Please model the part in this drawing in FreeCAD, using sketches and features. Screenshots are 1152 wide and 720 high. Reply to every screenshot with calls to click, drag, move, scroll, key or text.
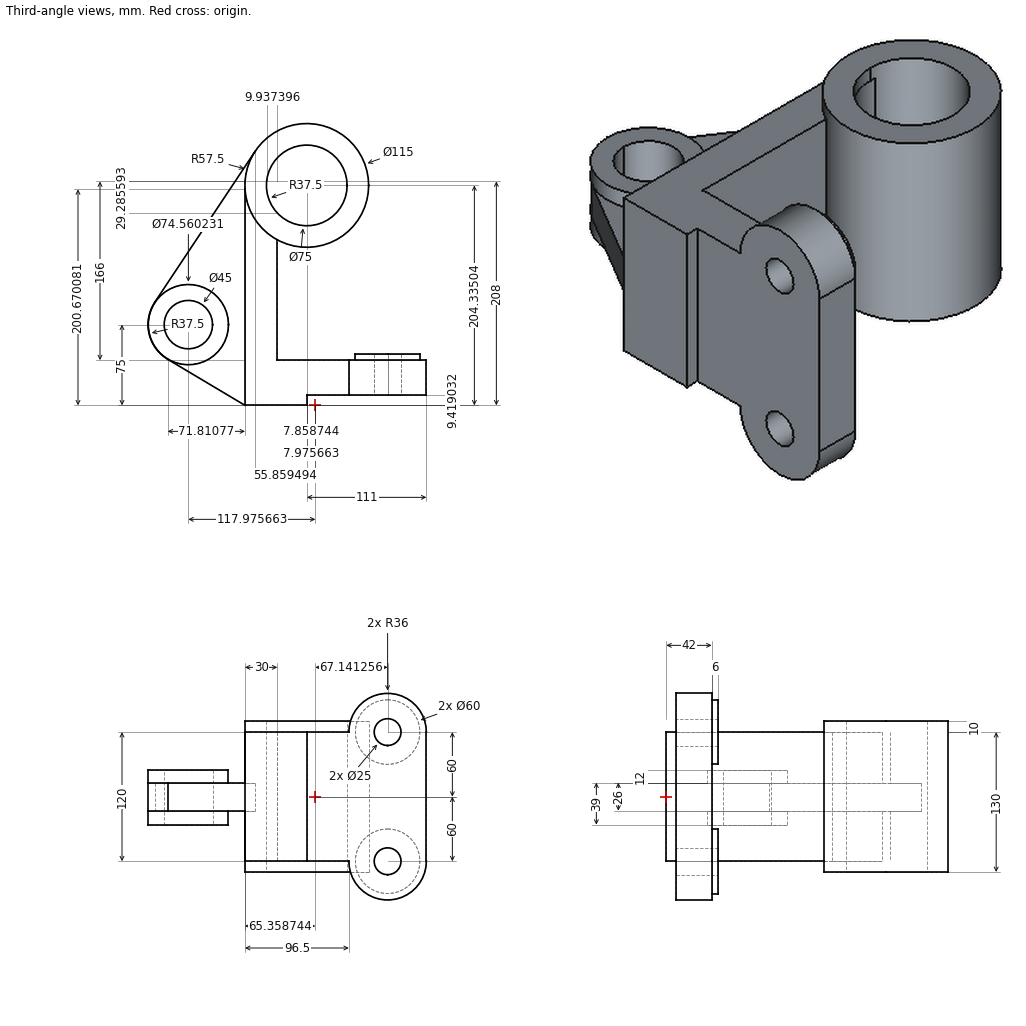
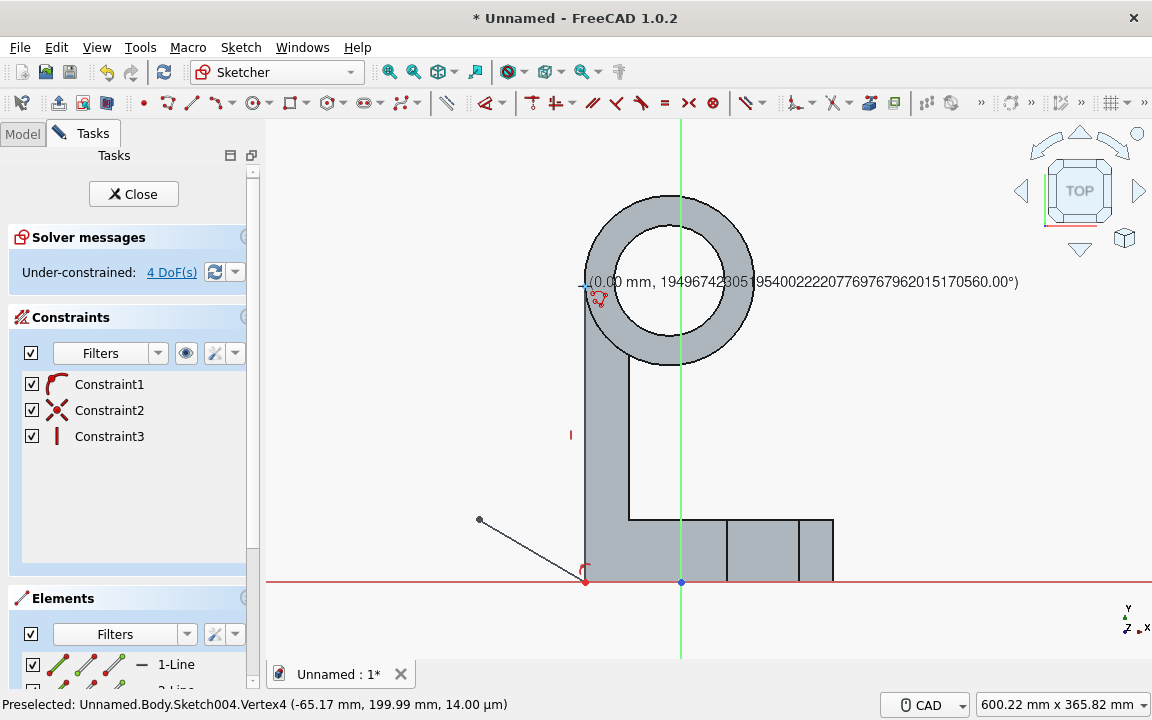
click(192, 104)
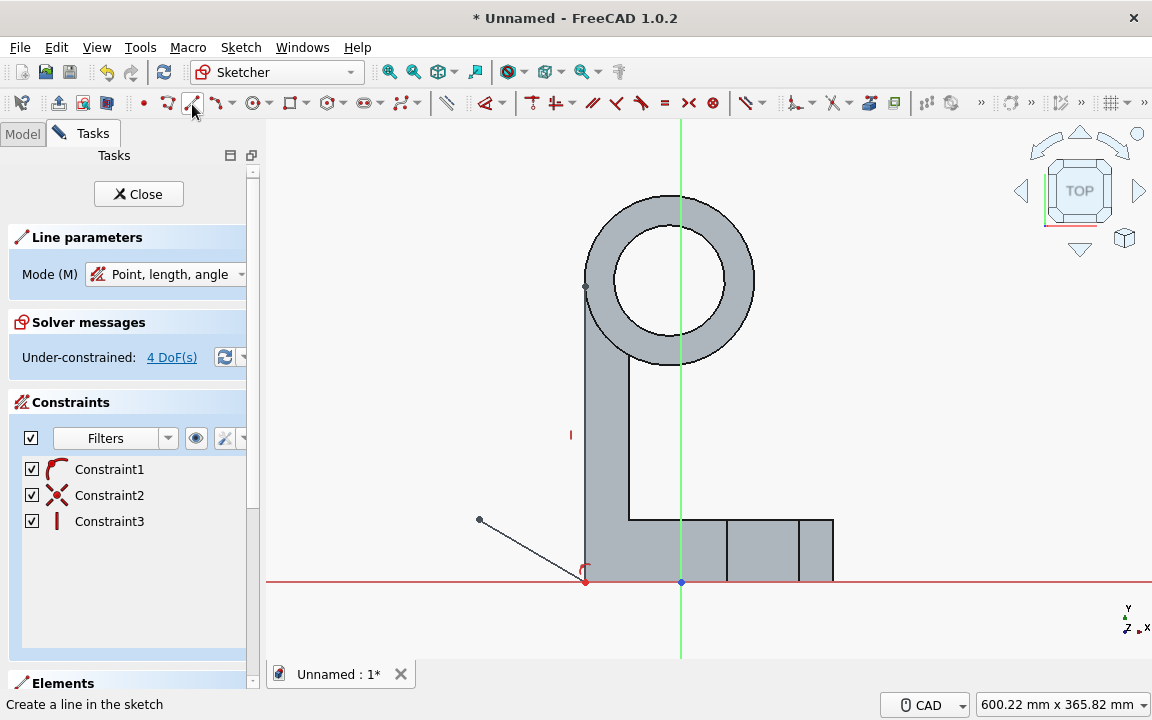
click(599, 234)
click(461, 441)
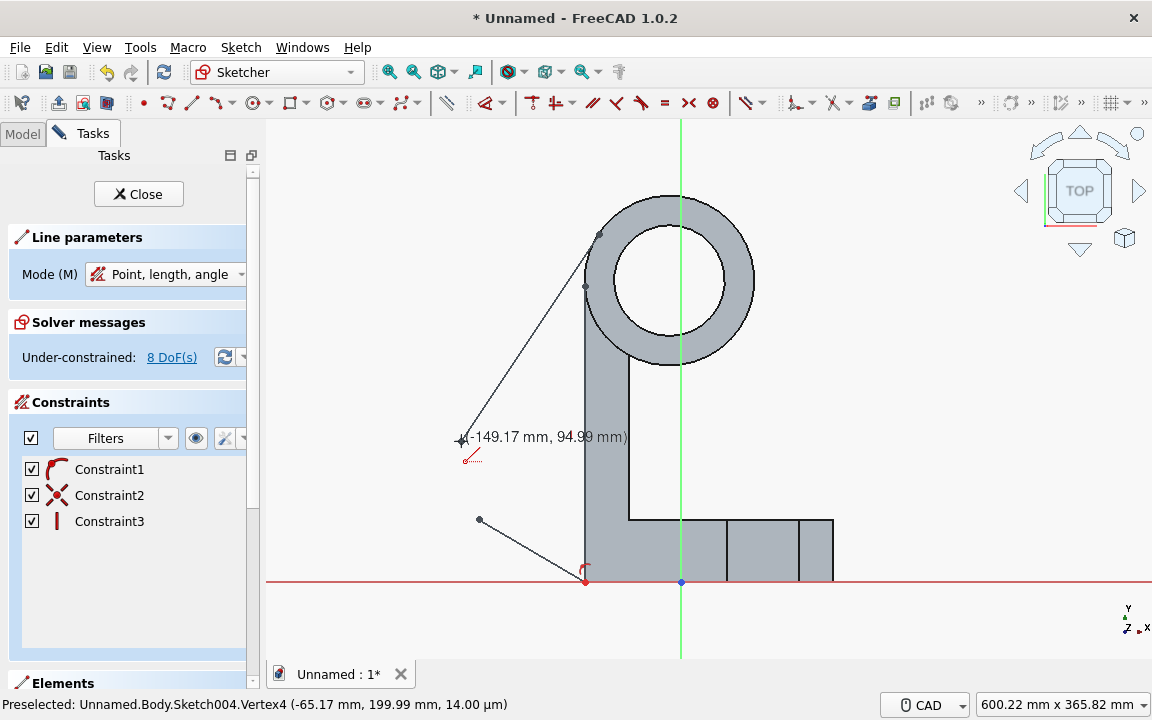
click(216, 104)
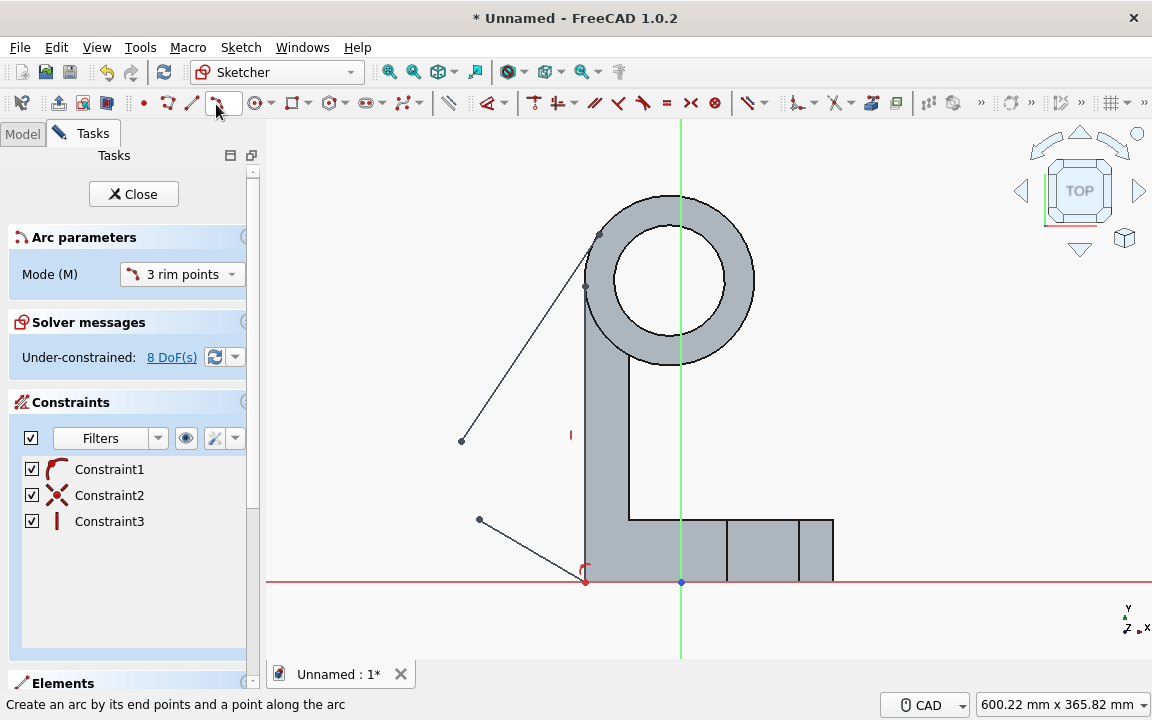
click(585, 287)
click(599, 235)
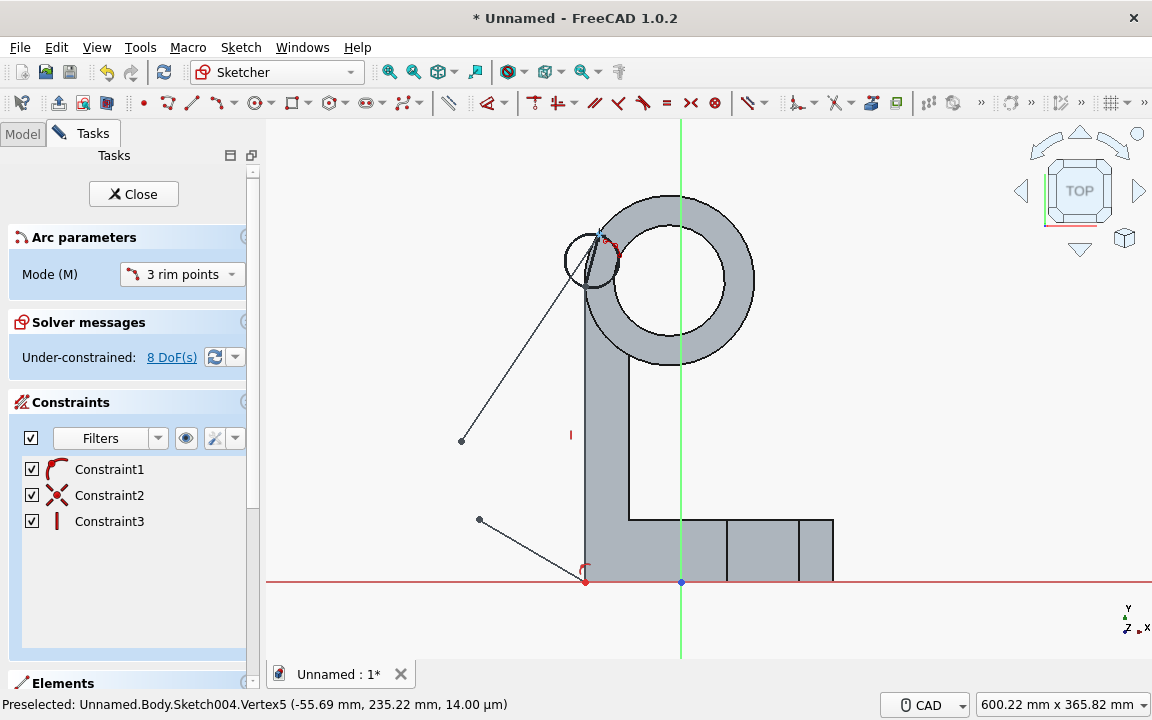
scroll(587, 259, up, 7)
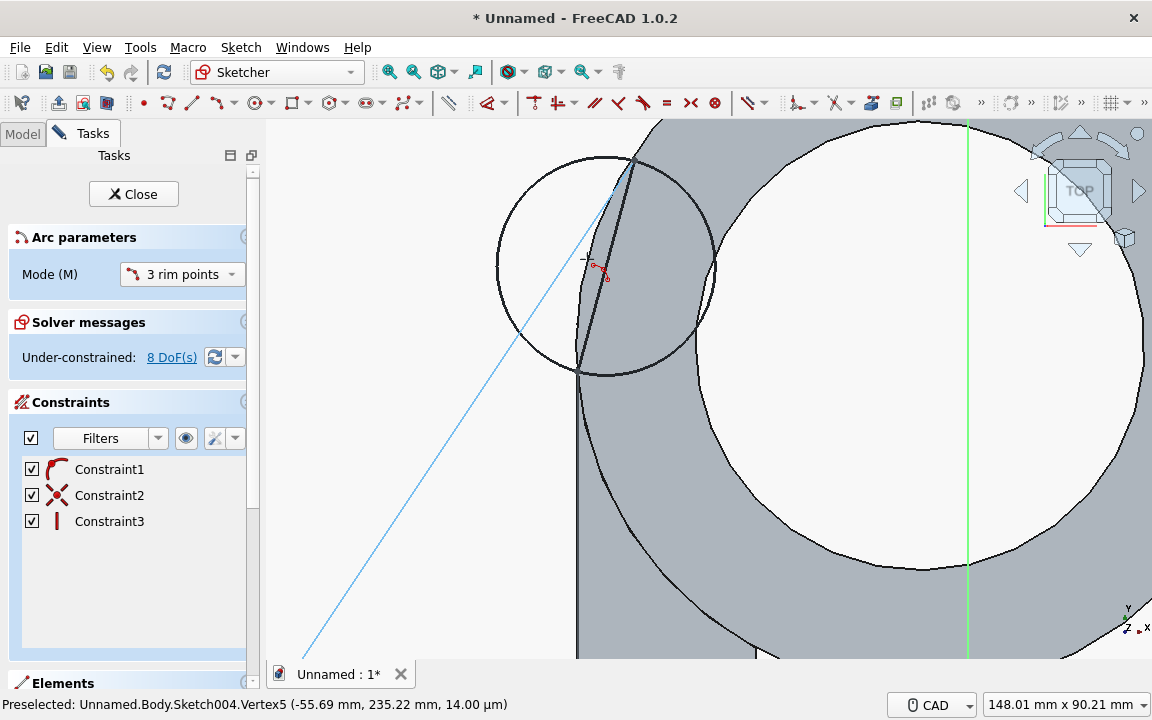
click(588, 257)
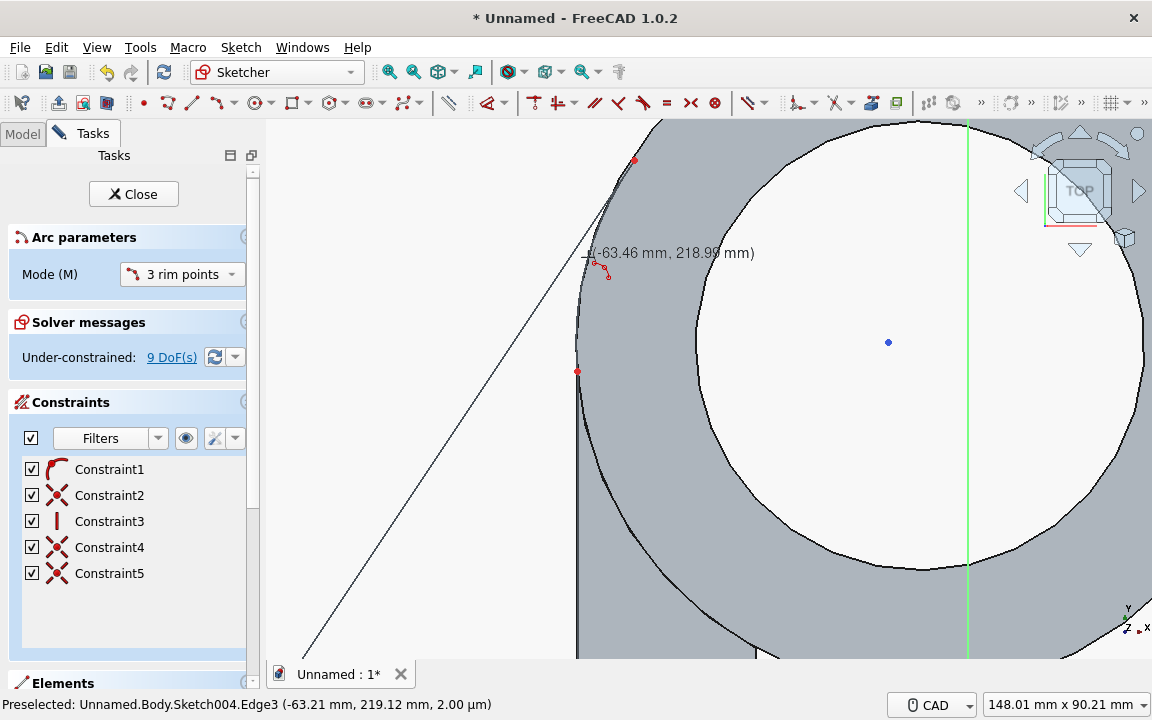
scroll(685, 234, down, 7)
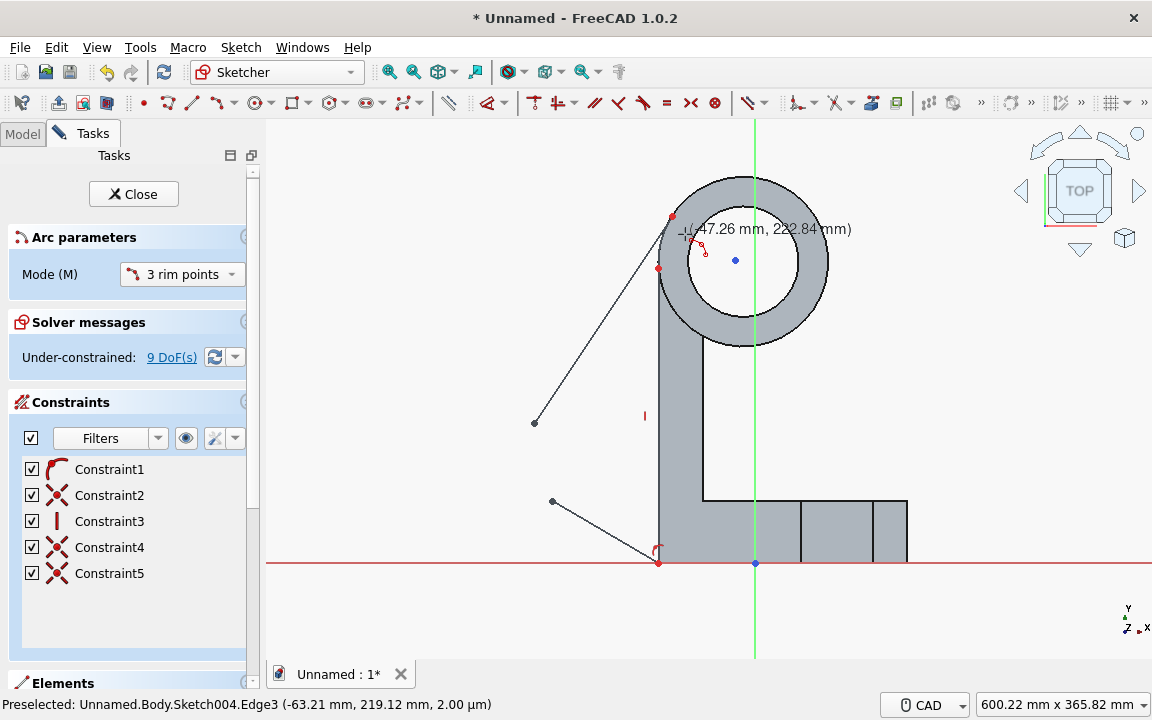
click(535, 423)
click(553, 501)
click(527, 465)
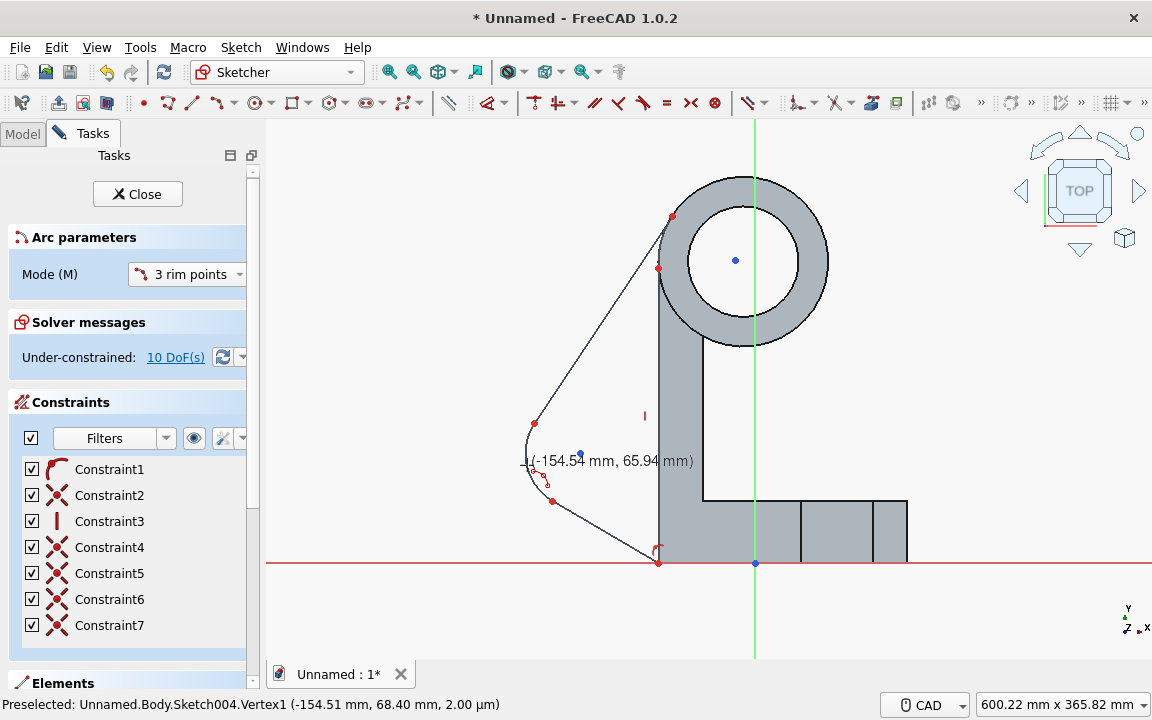
click(256, 104)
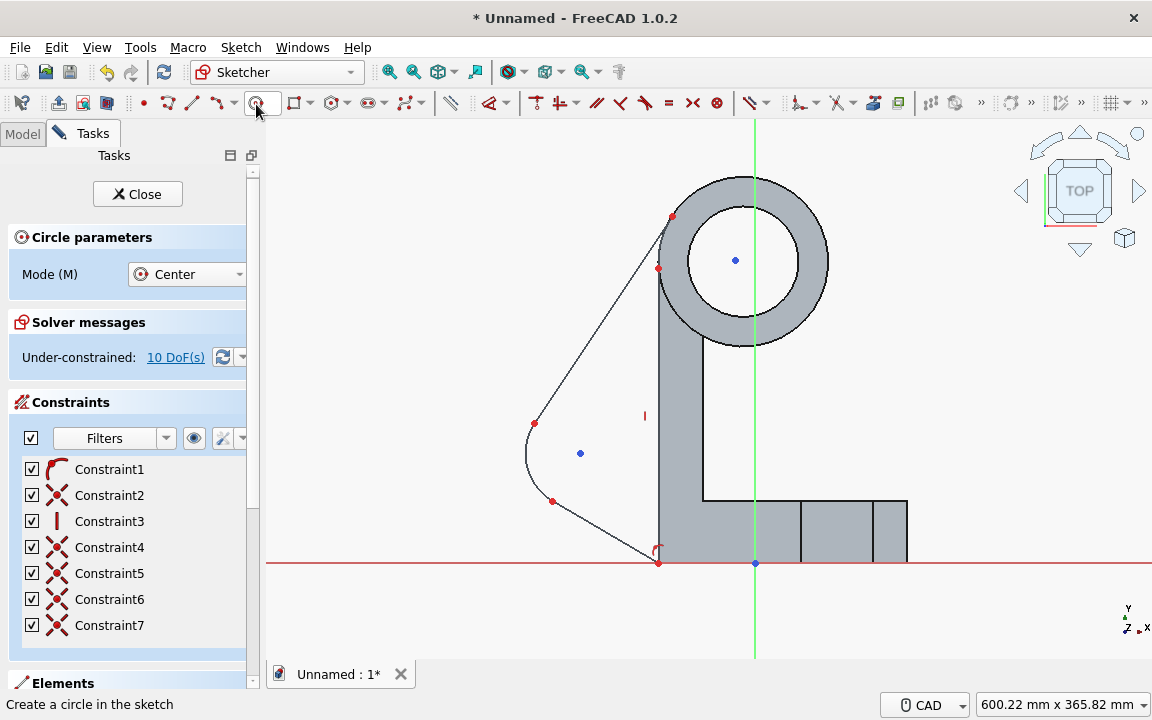
click(581, 453)
move(604, 429)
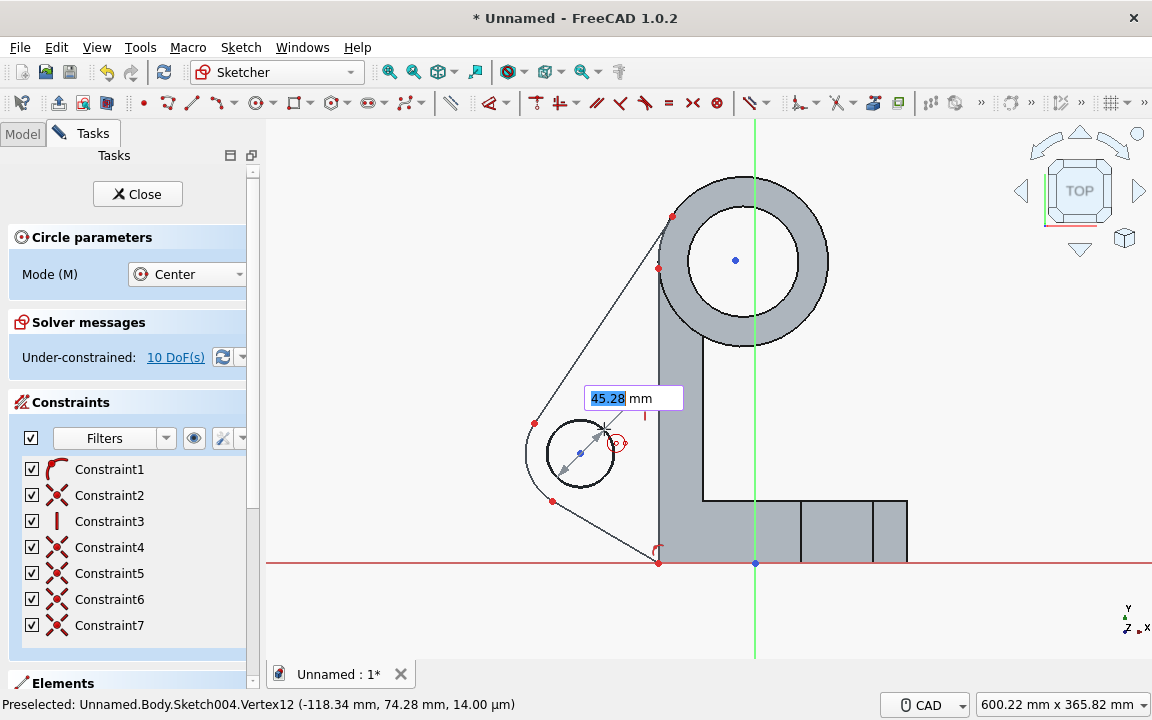
text(45)
key(Return)
key(Escape)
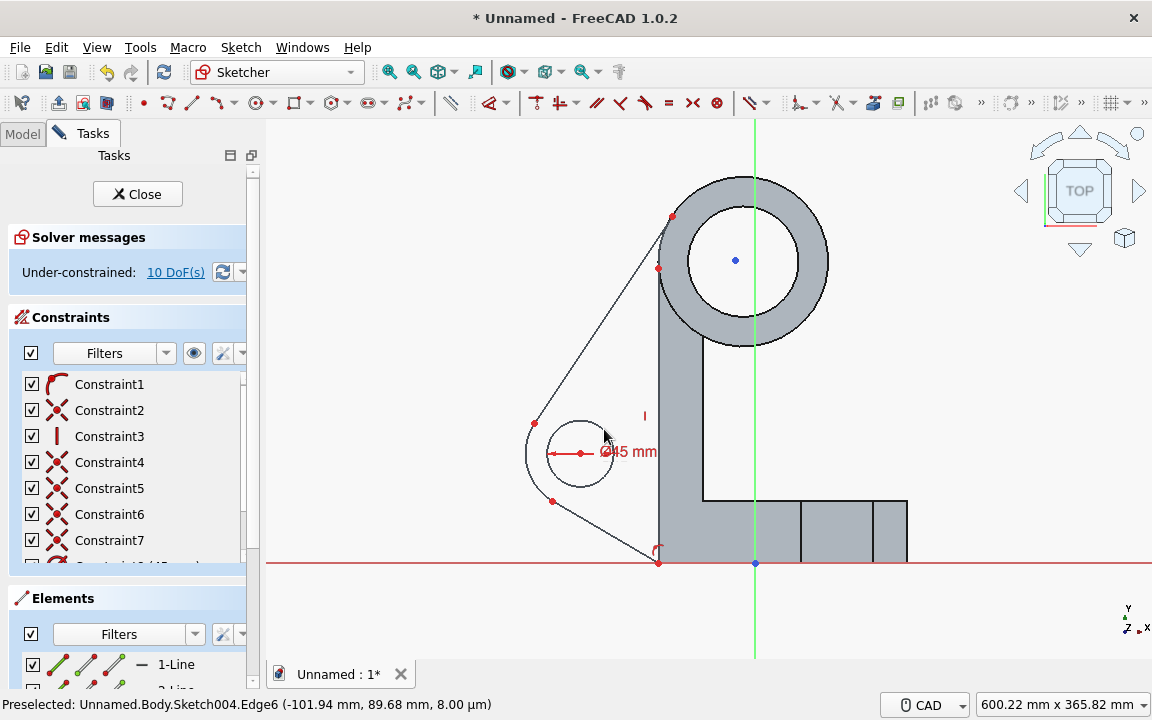
click(585, 520)